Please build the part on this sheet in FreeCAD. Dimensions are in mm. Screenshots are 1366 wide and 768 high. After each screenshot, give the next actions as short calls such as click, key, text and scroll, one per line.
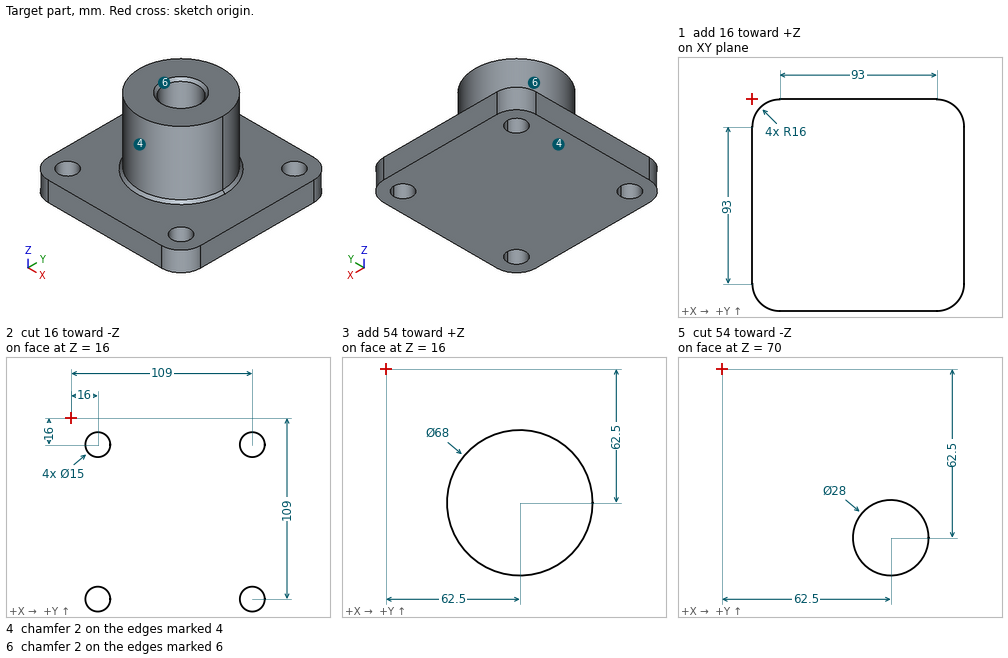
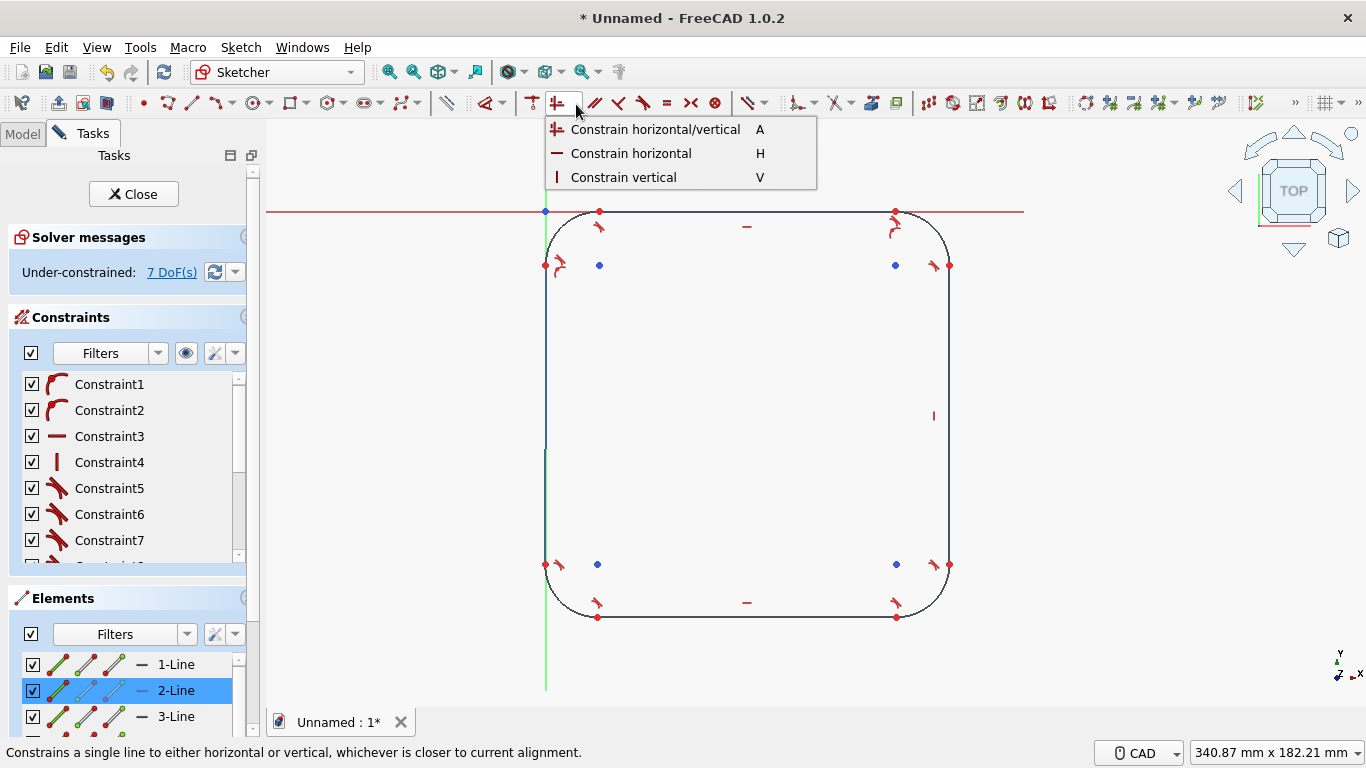
click(681, 177)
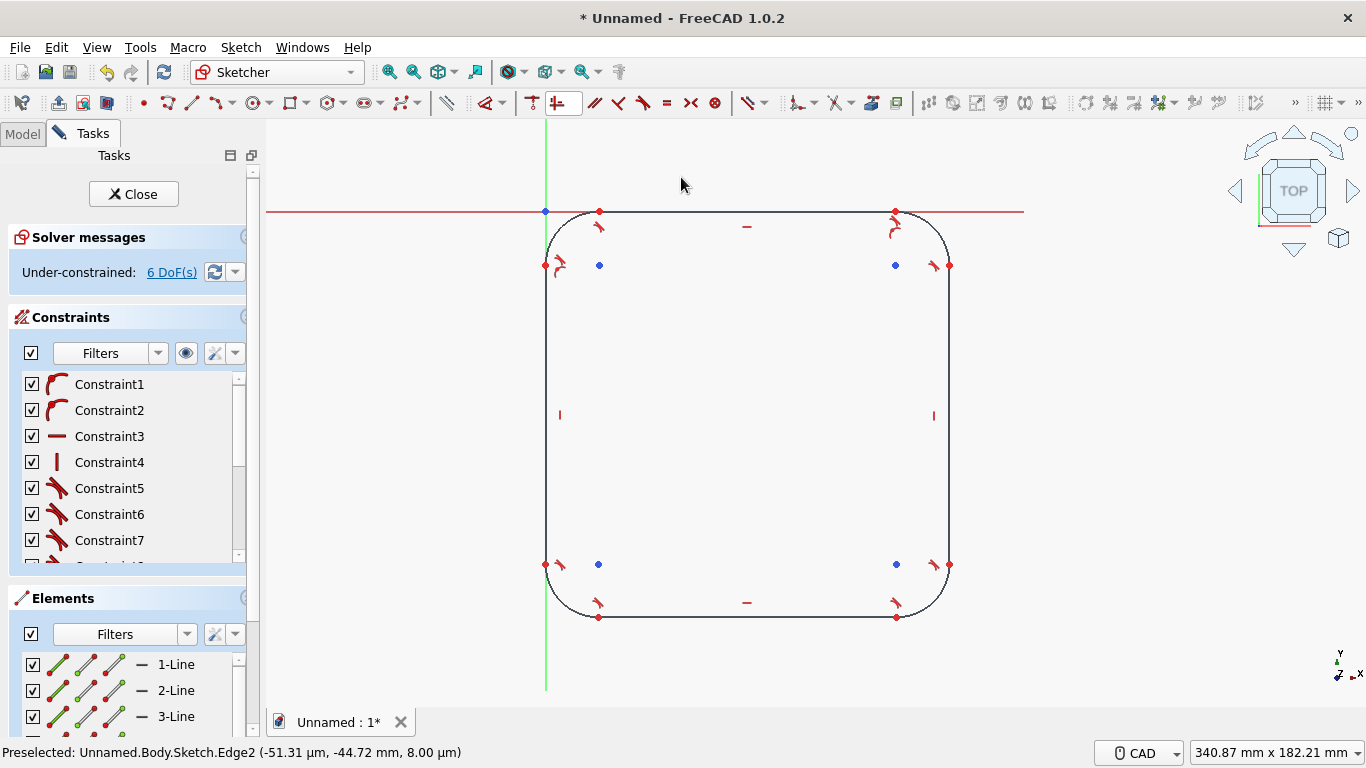
click(561, 227)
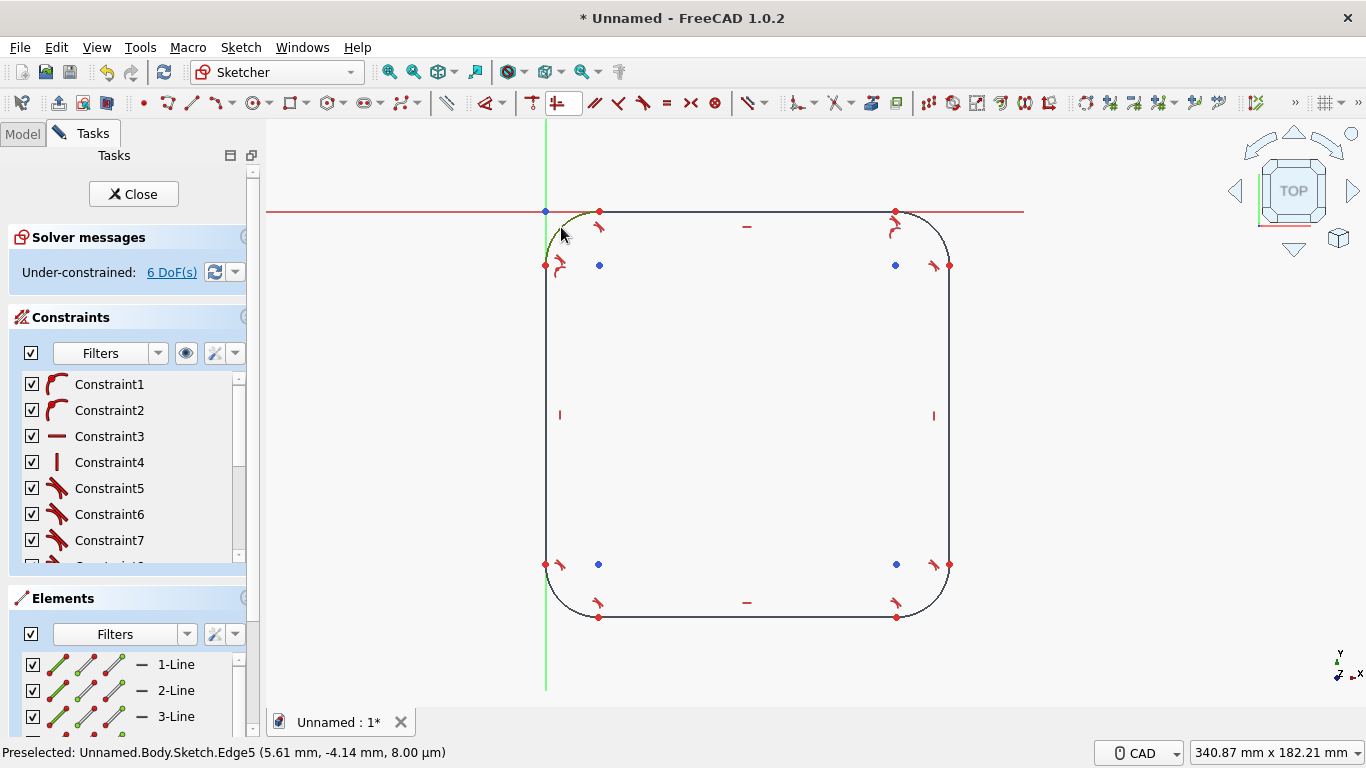
click(574, 611)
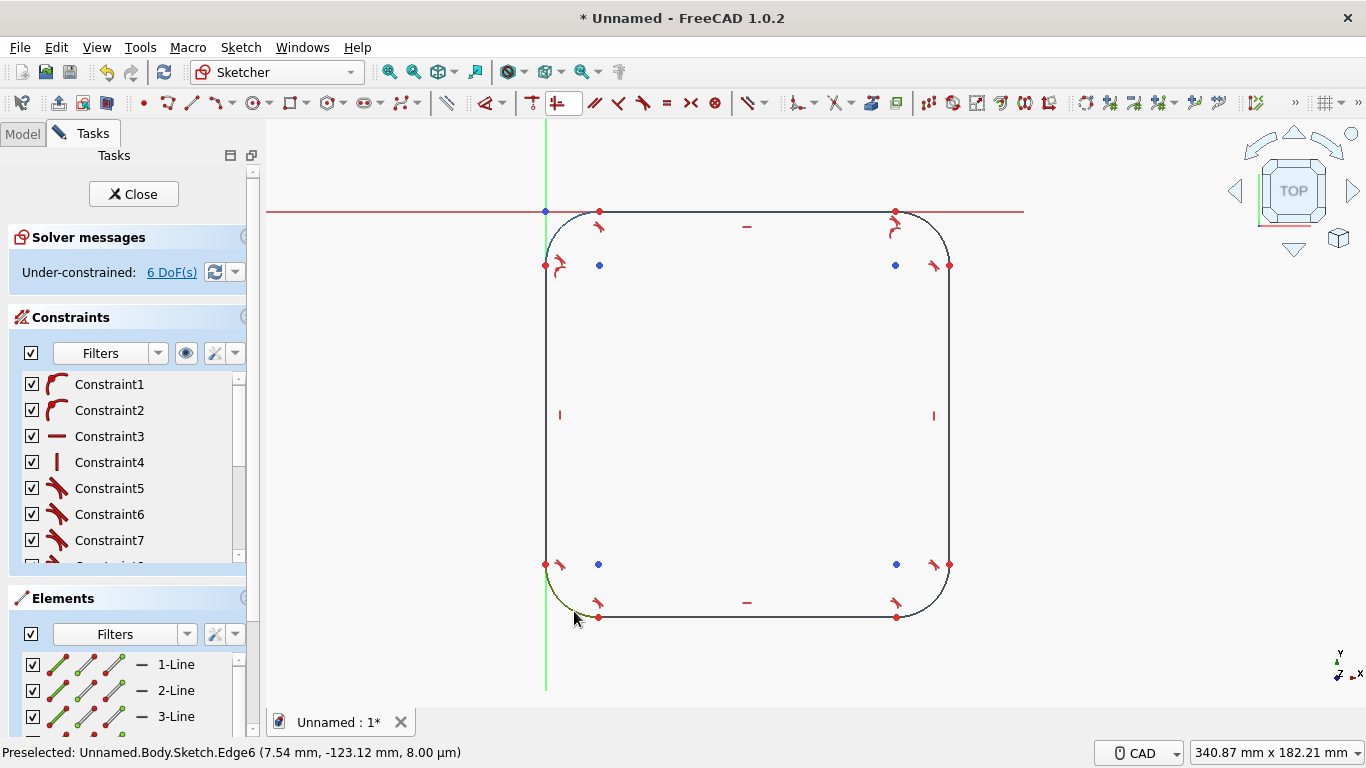
click(920, 611)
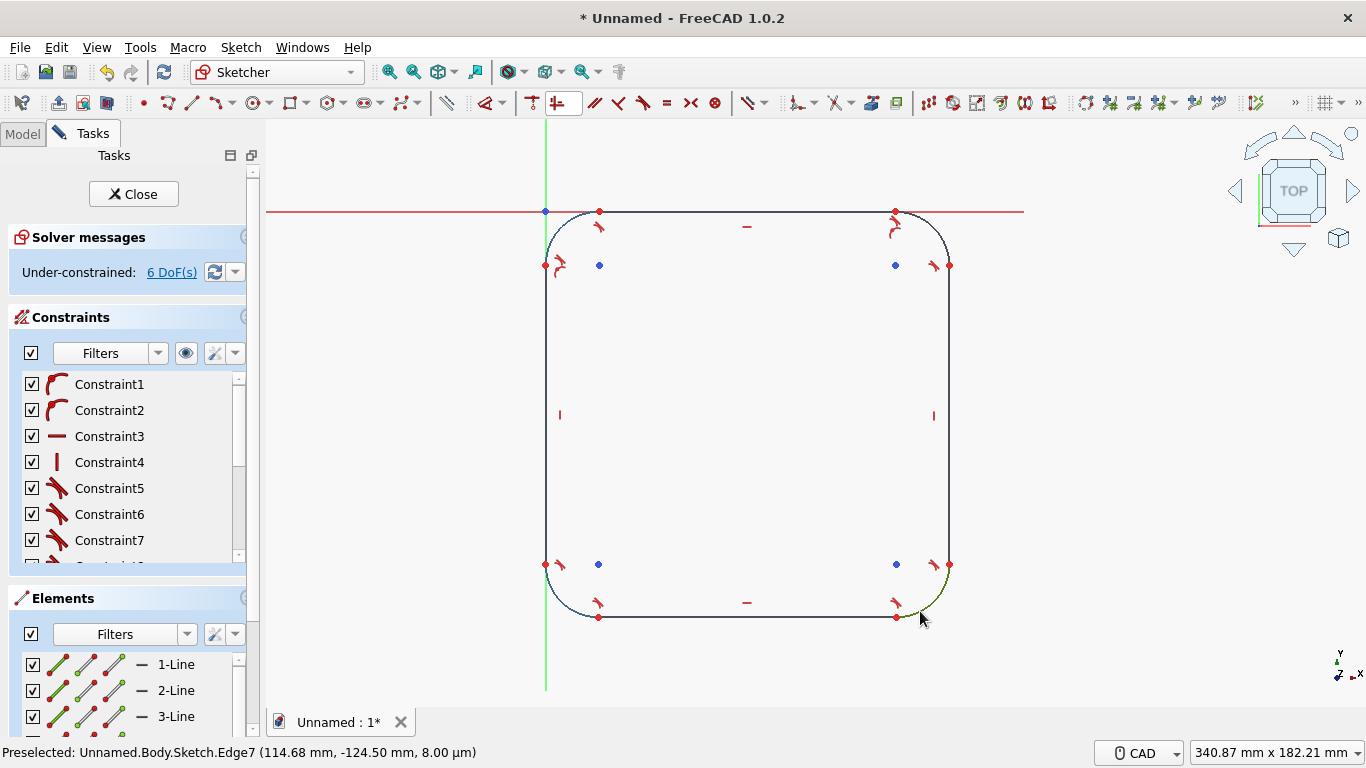
click(943, 241)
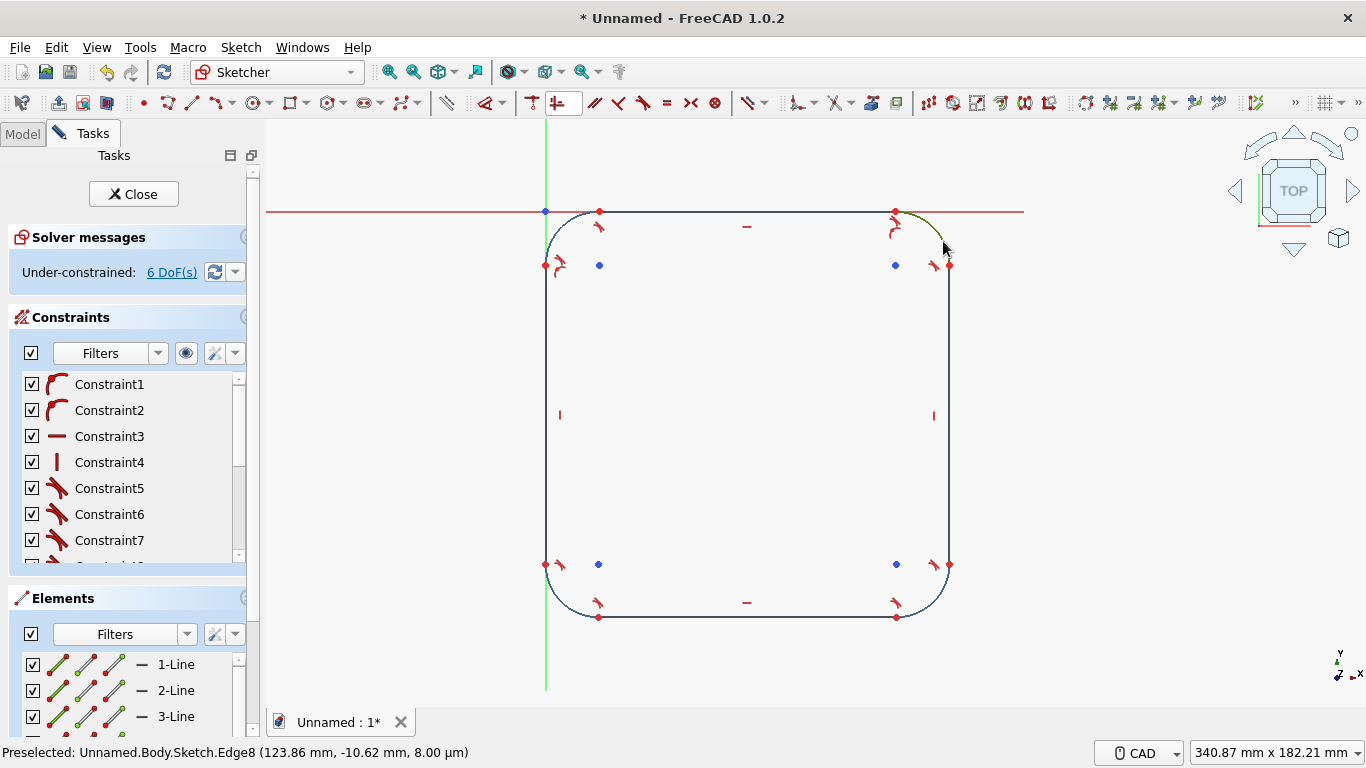
key(e)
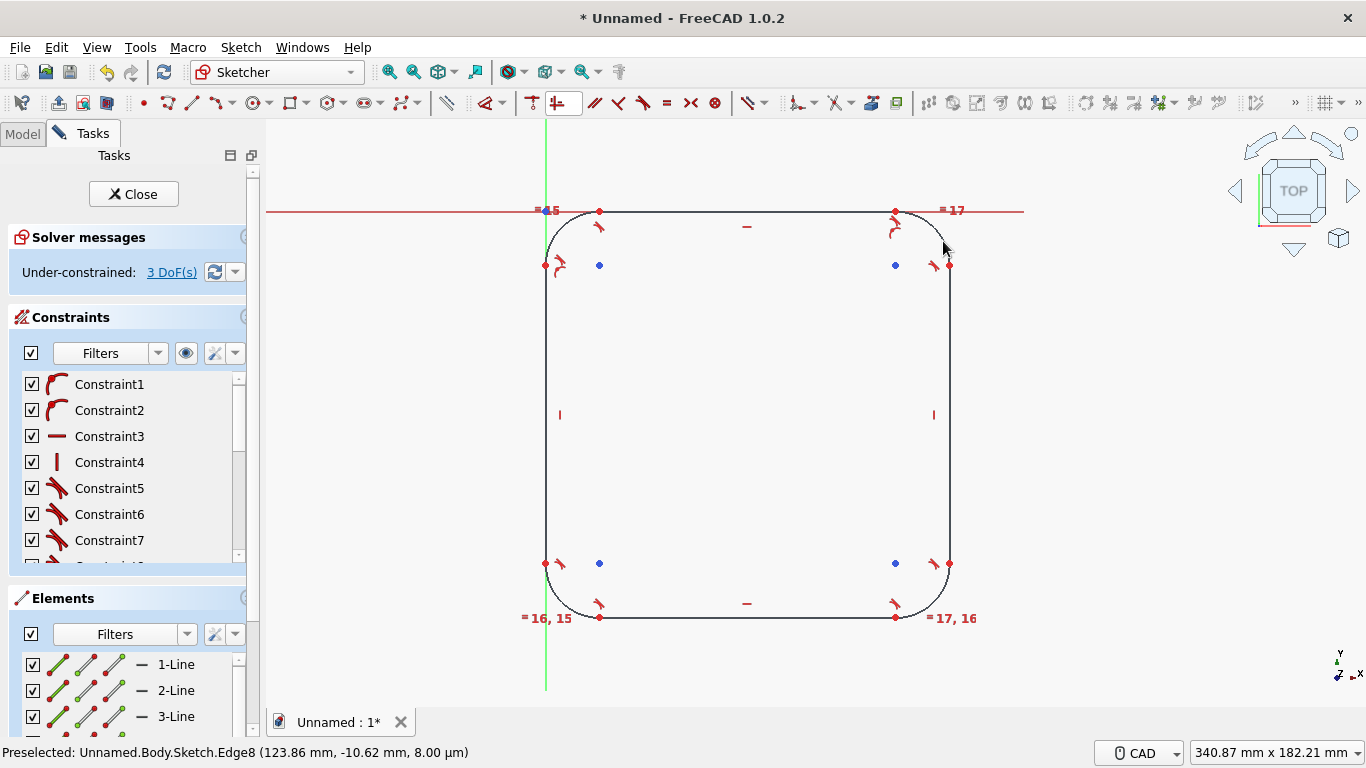
key(d)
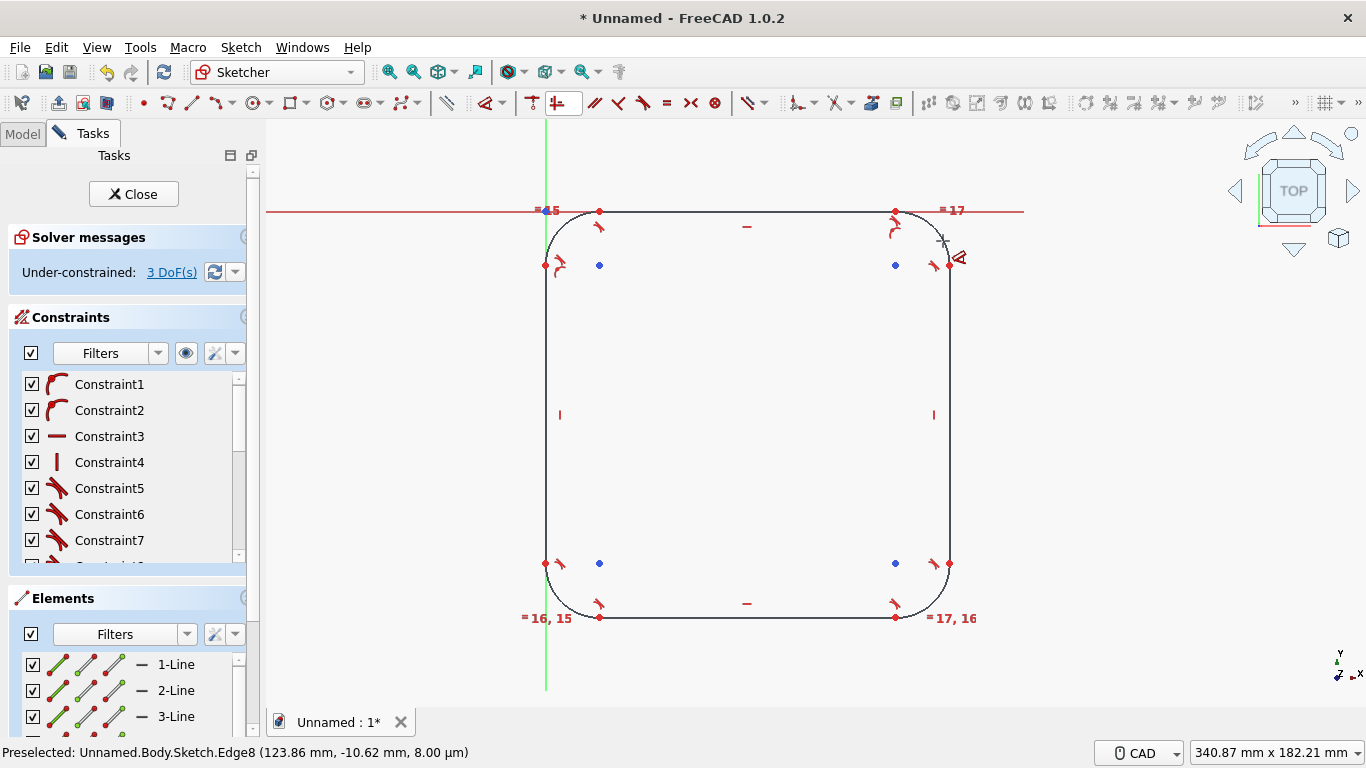
click(562, 228)
click(576, 184)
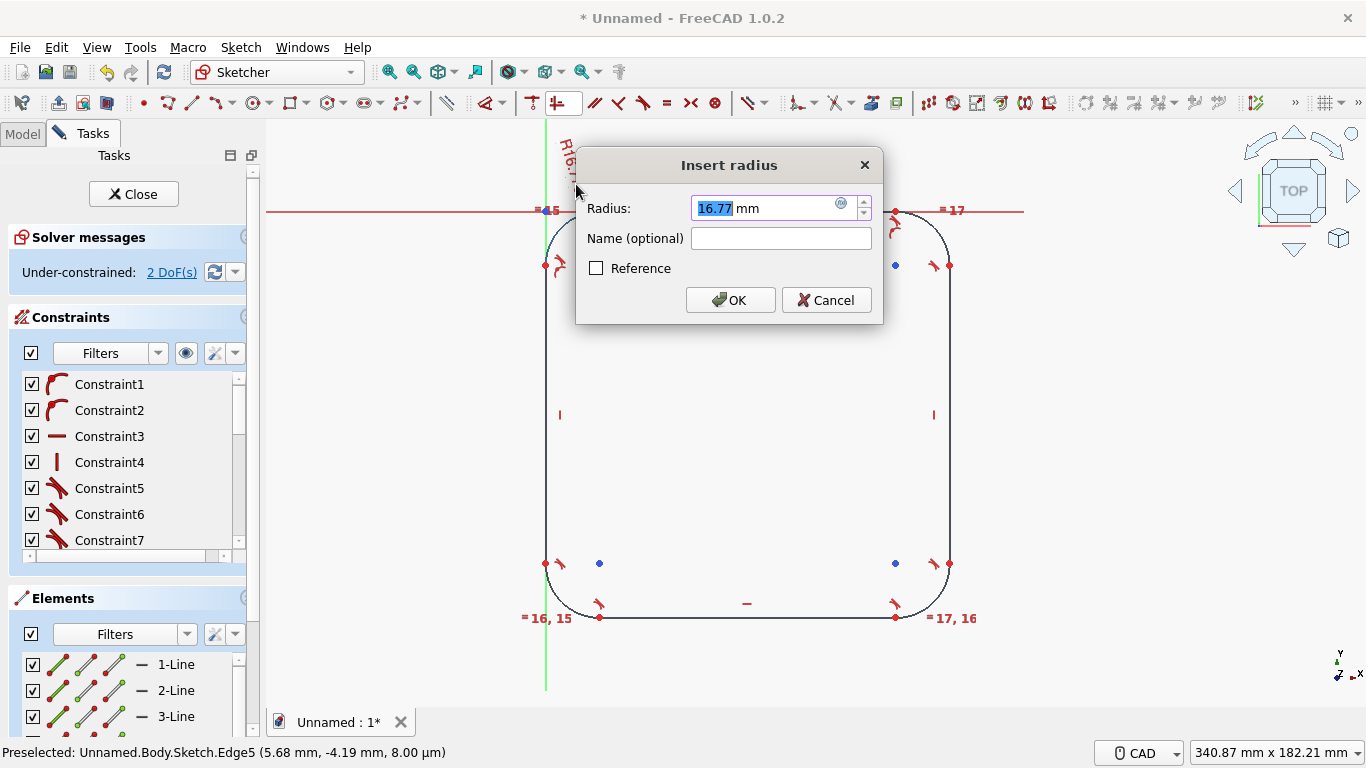
text(16)
key(Return)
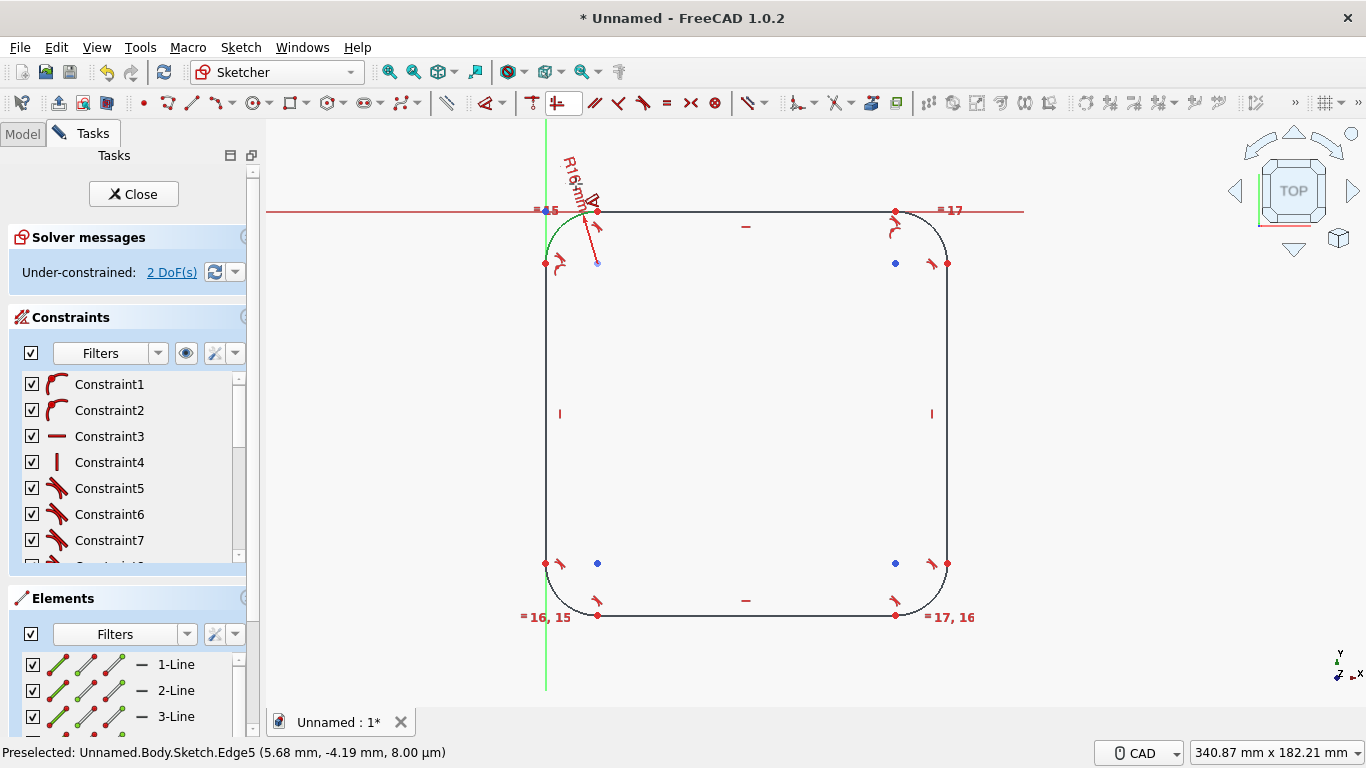
click(806, 212)
click(747, 178)